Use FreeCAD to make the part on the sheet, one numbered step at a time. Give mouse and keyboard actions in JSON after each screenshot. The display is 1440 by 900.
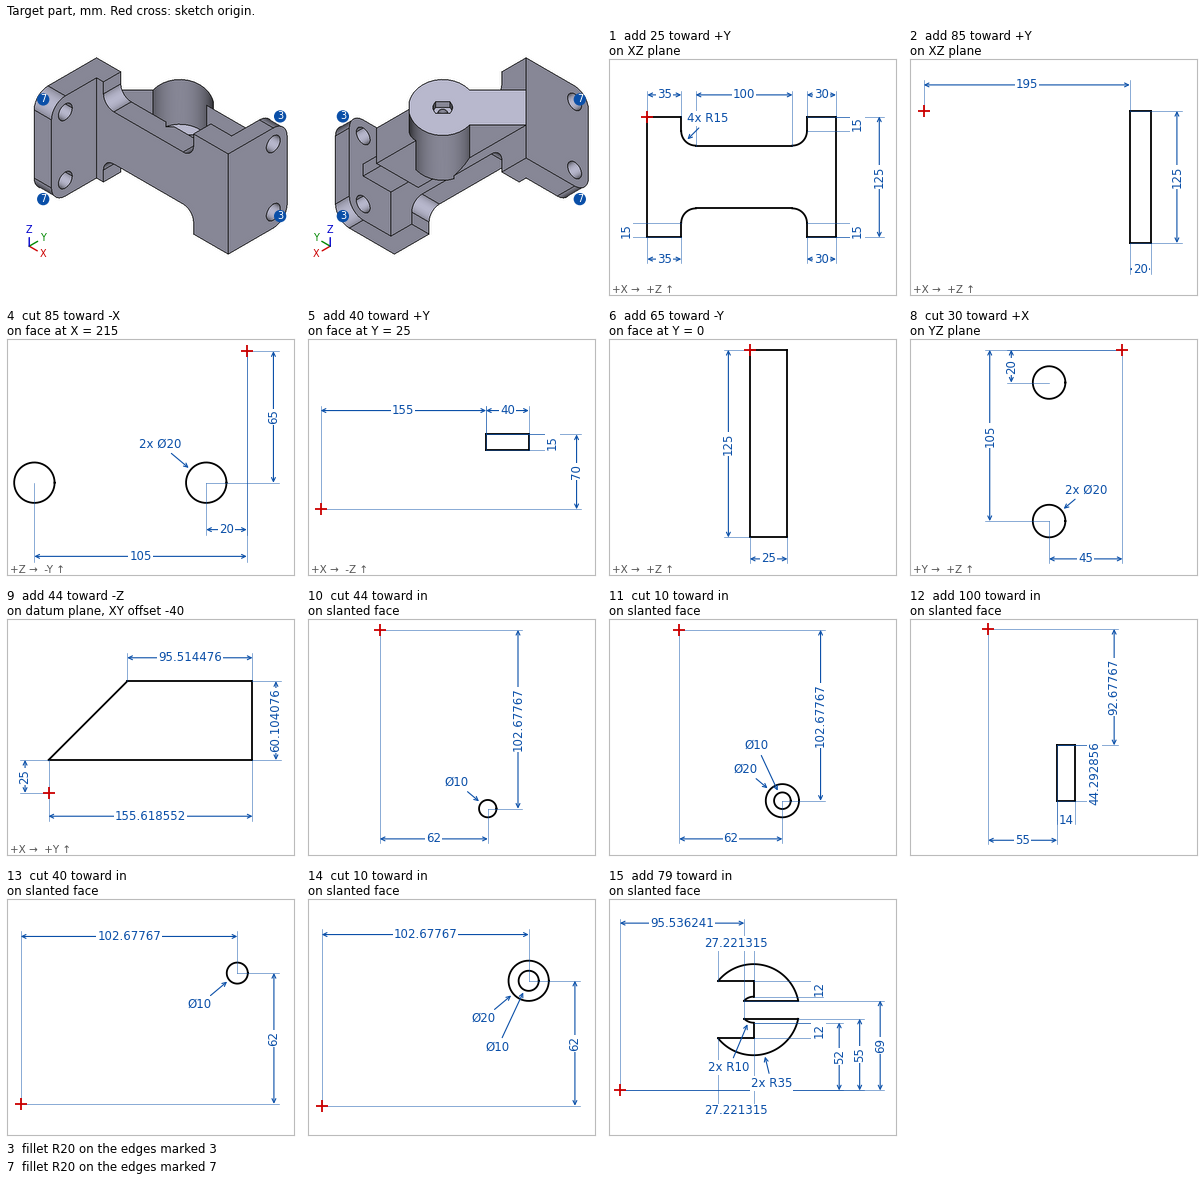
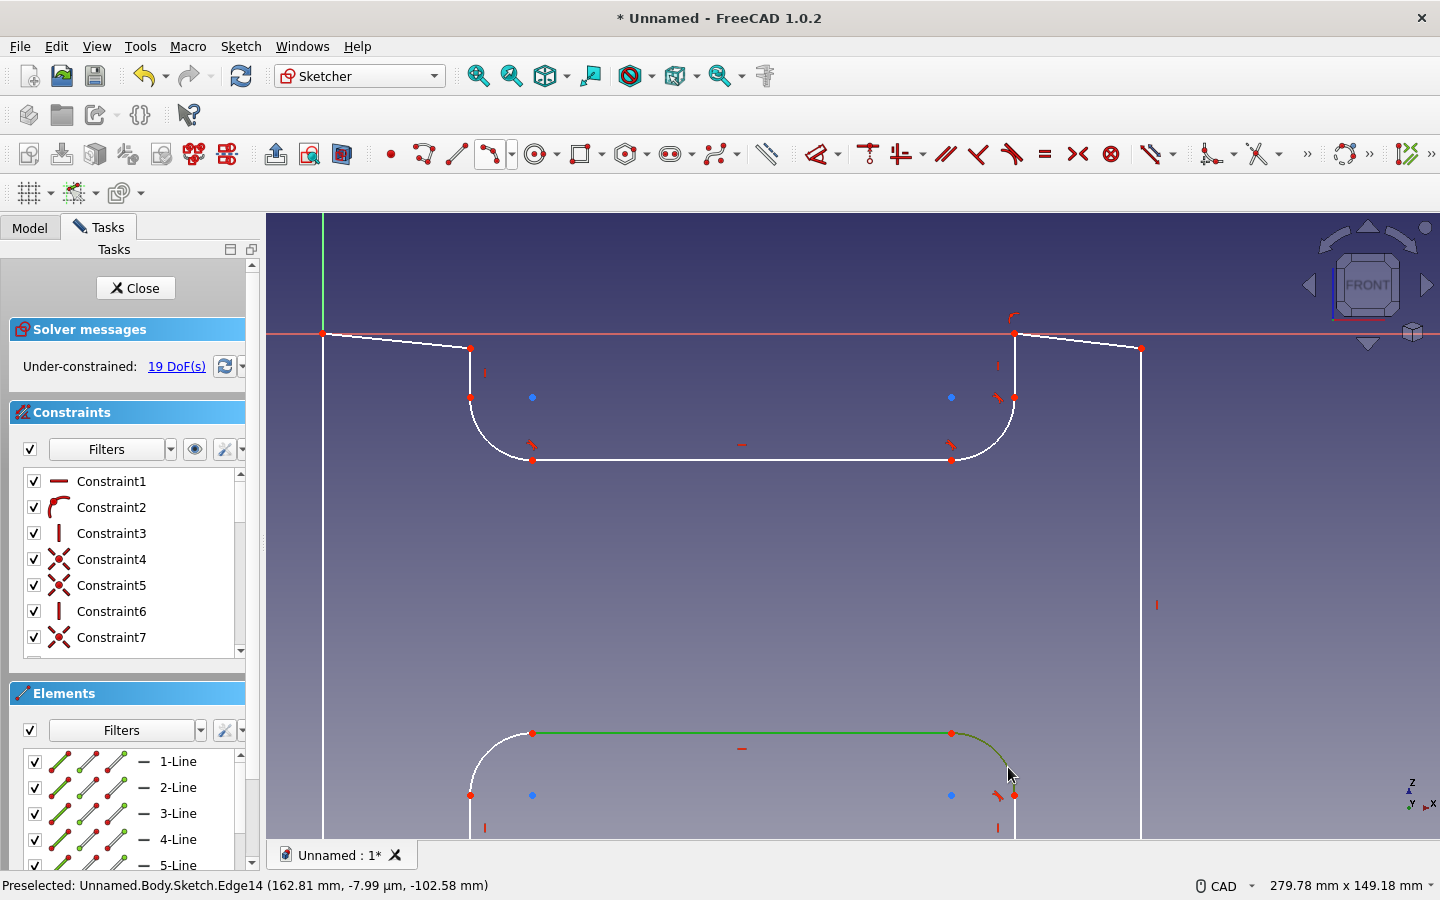
{"action": "left_click", "coordinate": [1012, 154]}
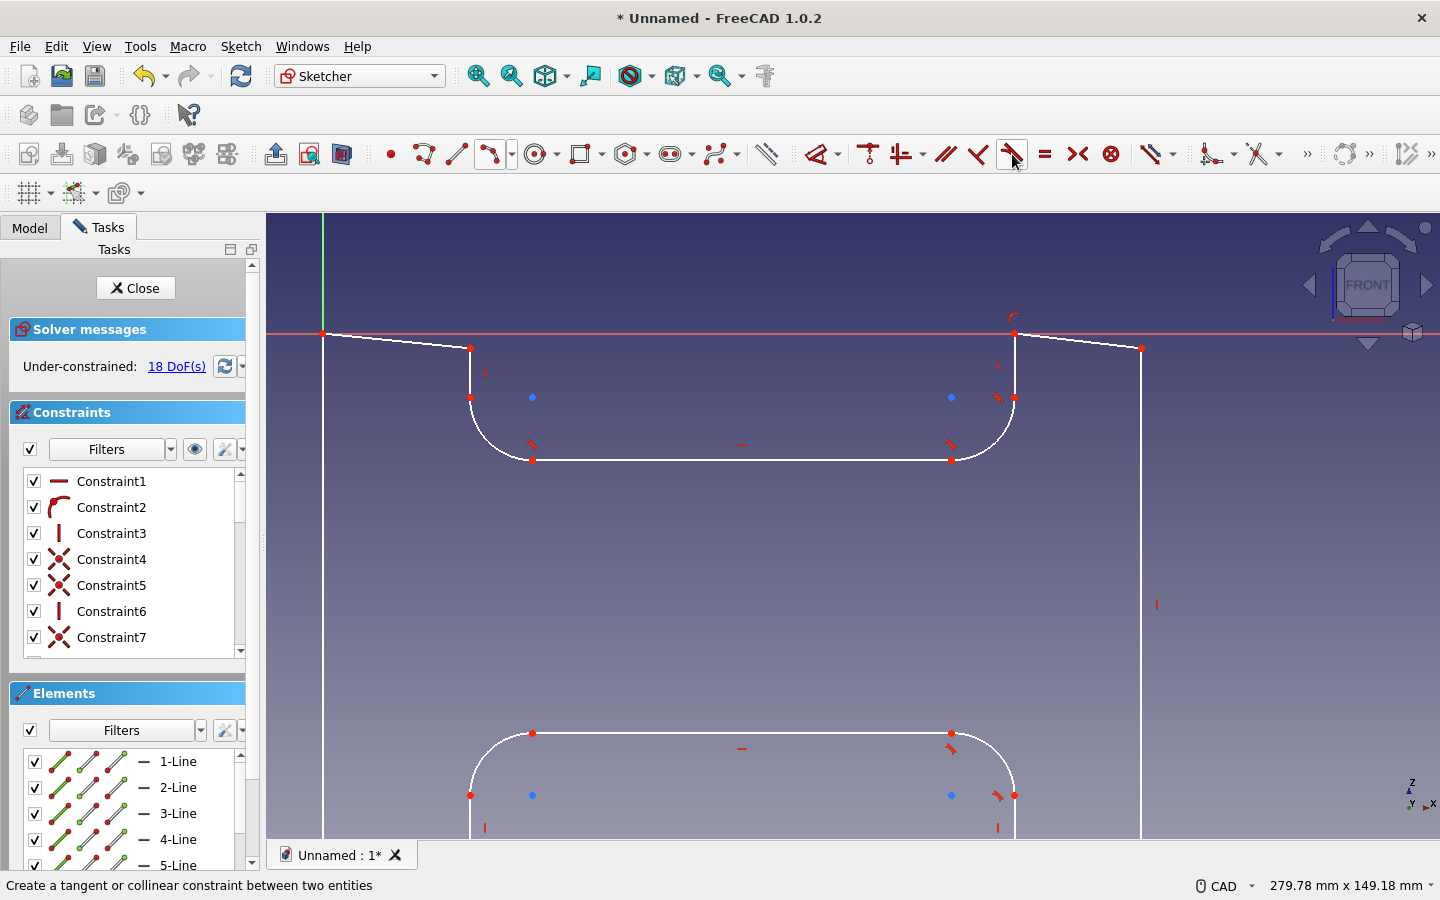
{"action": "left_click", "coordinate": [826, 733]}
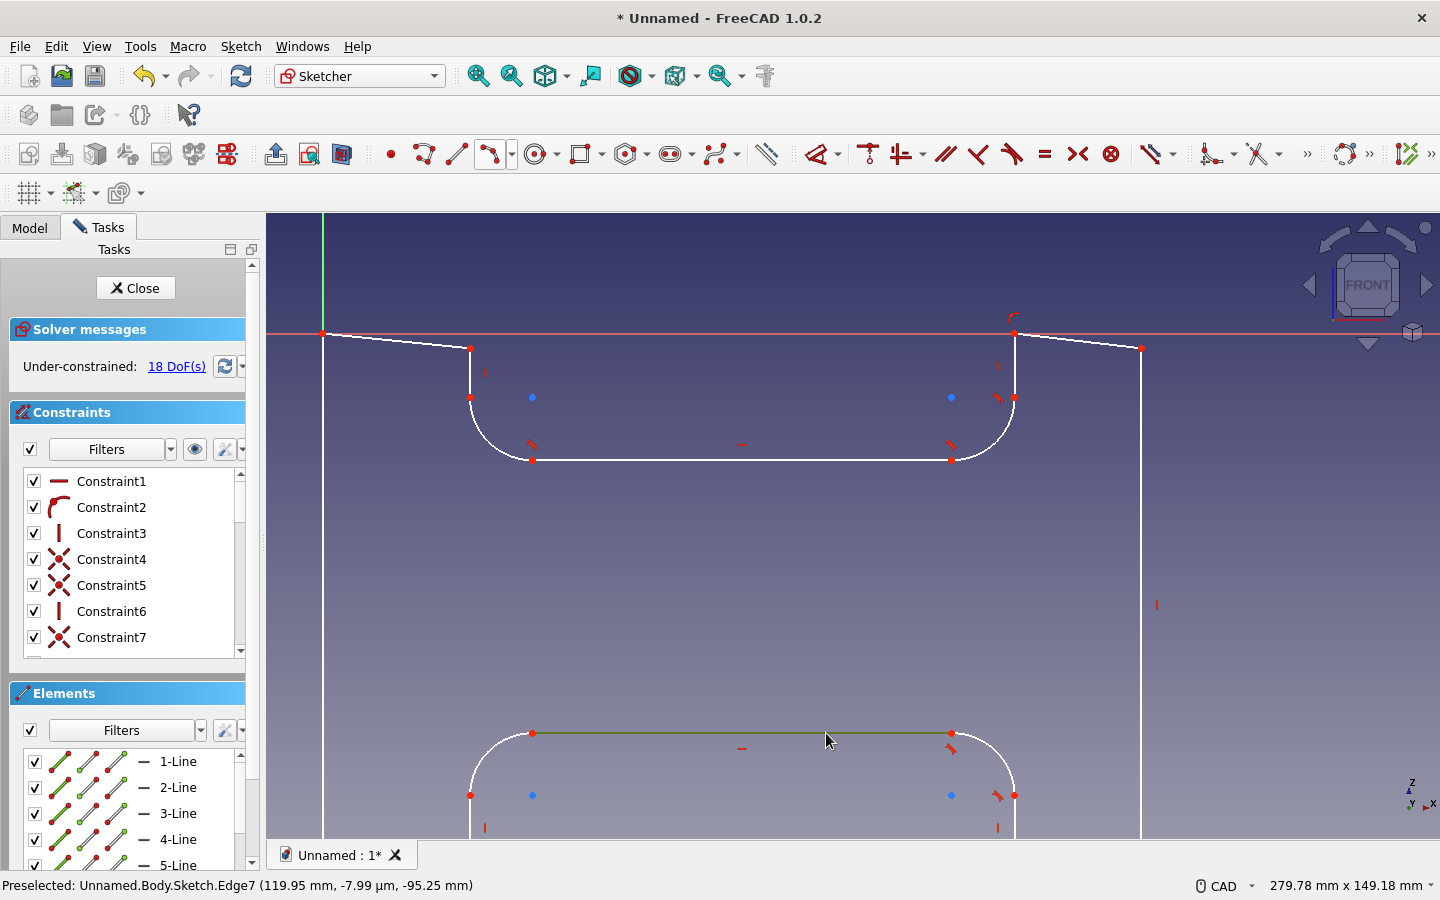
{"action": "left_click", "coordinate": [504, 740]}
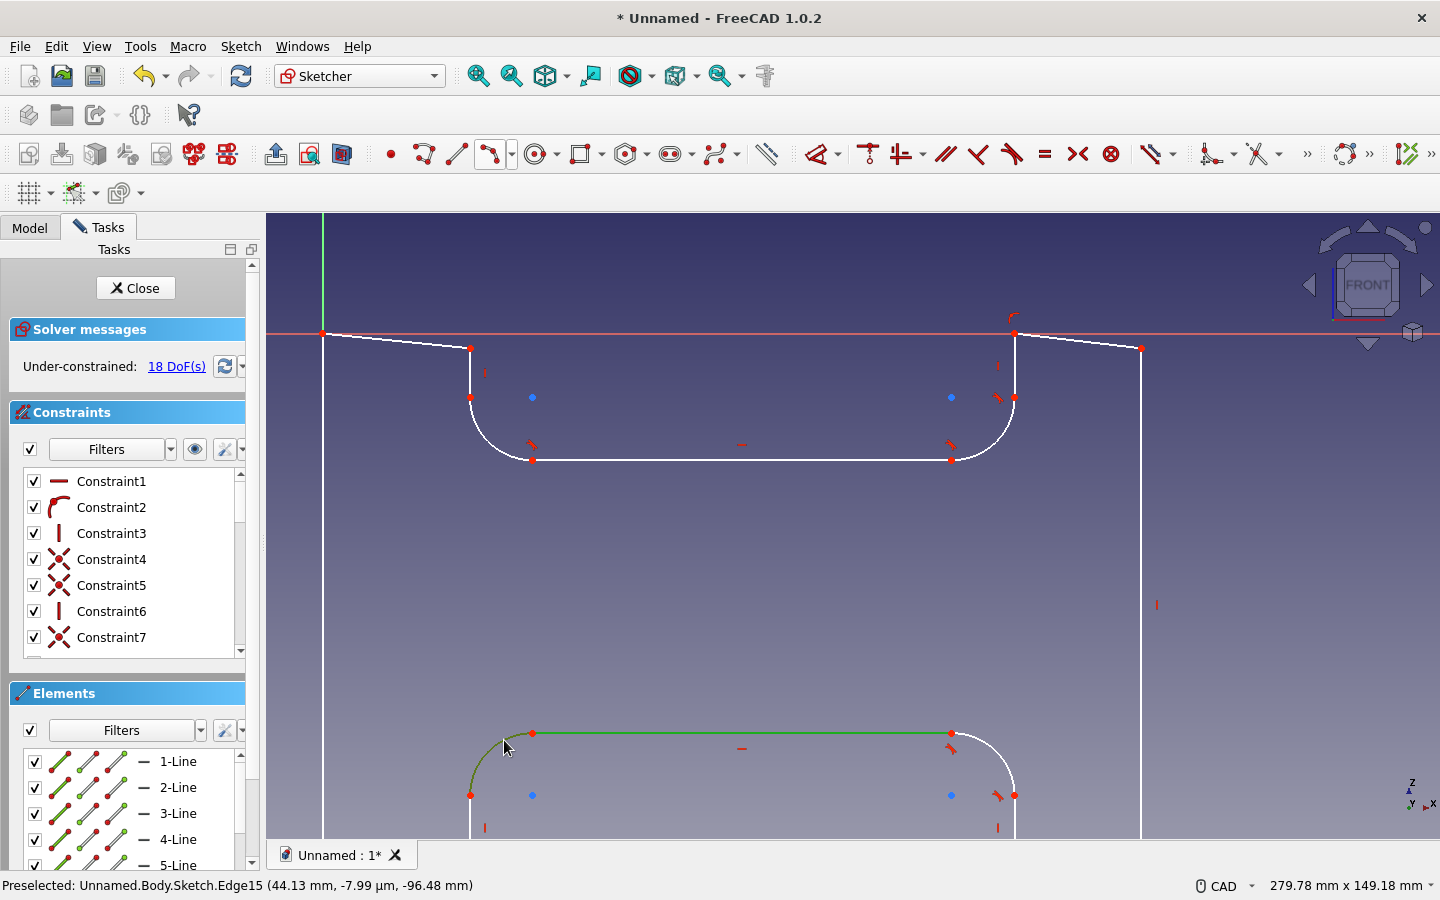
{"action": "left_click", "coordinate": [1012, 154]}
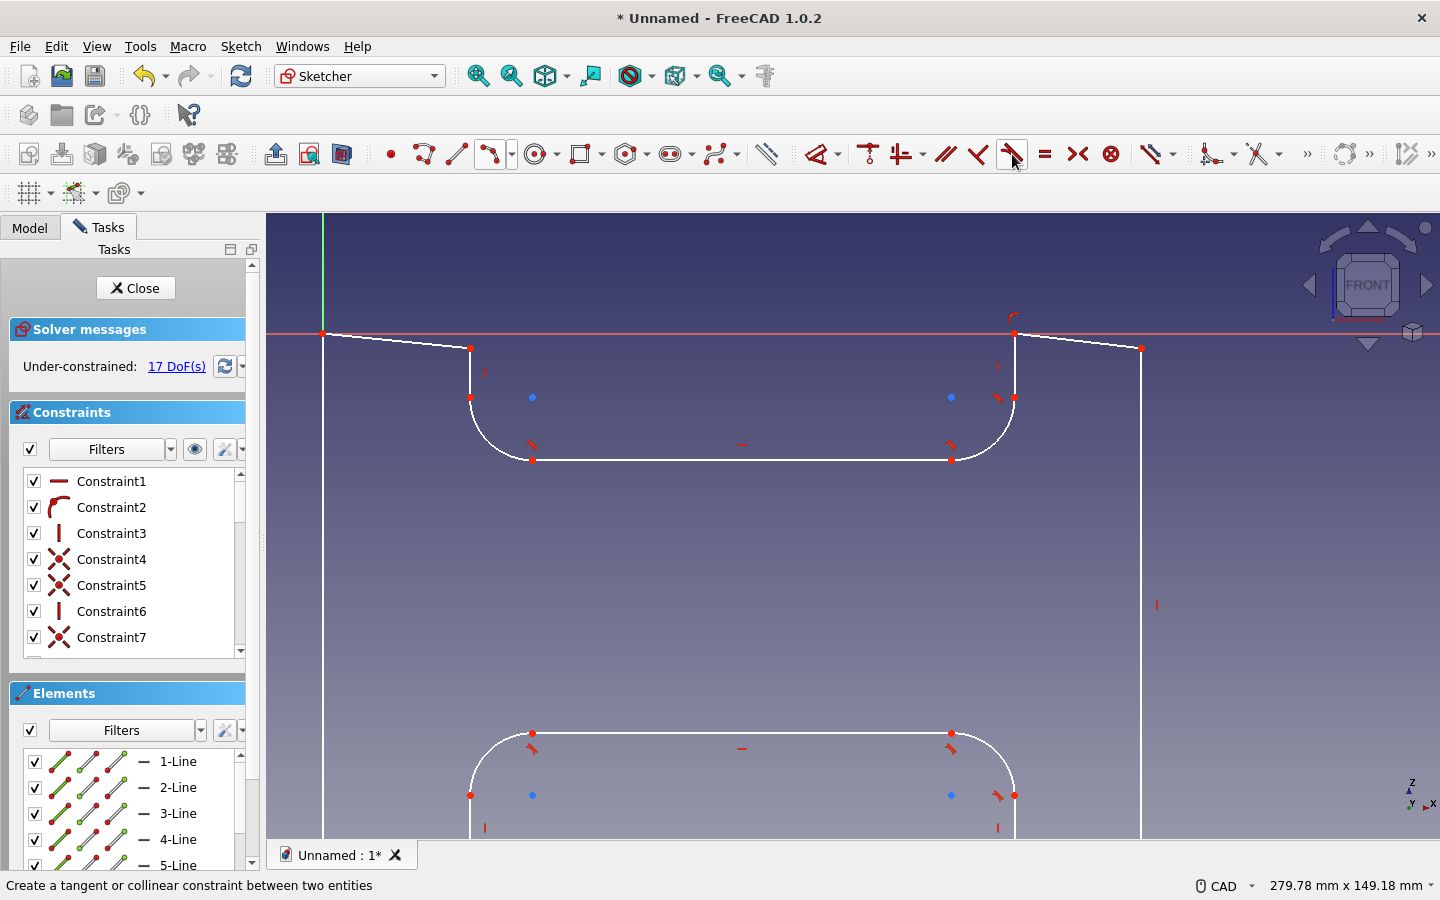
{"action": "left_click", "coordinate": [470, 809]}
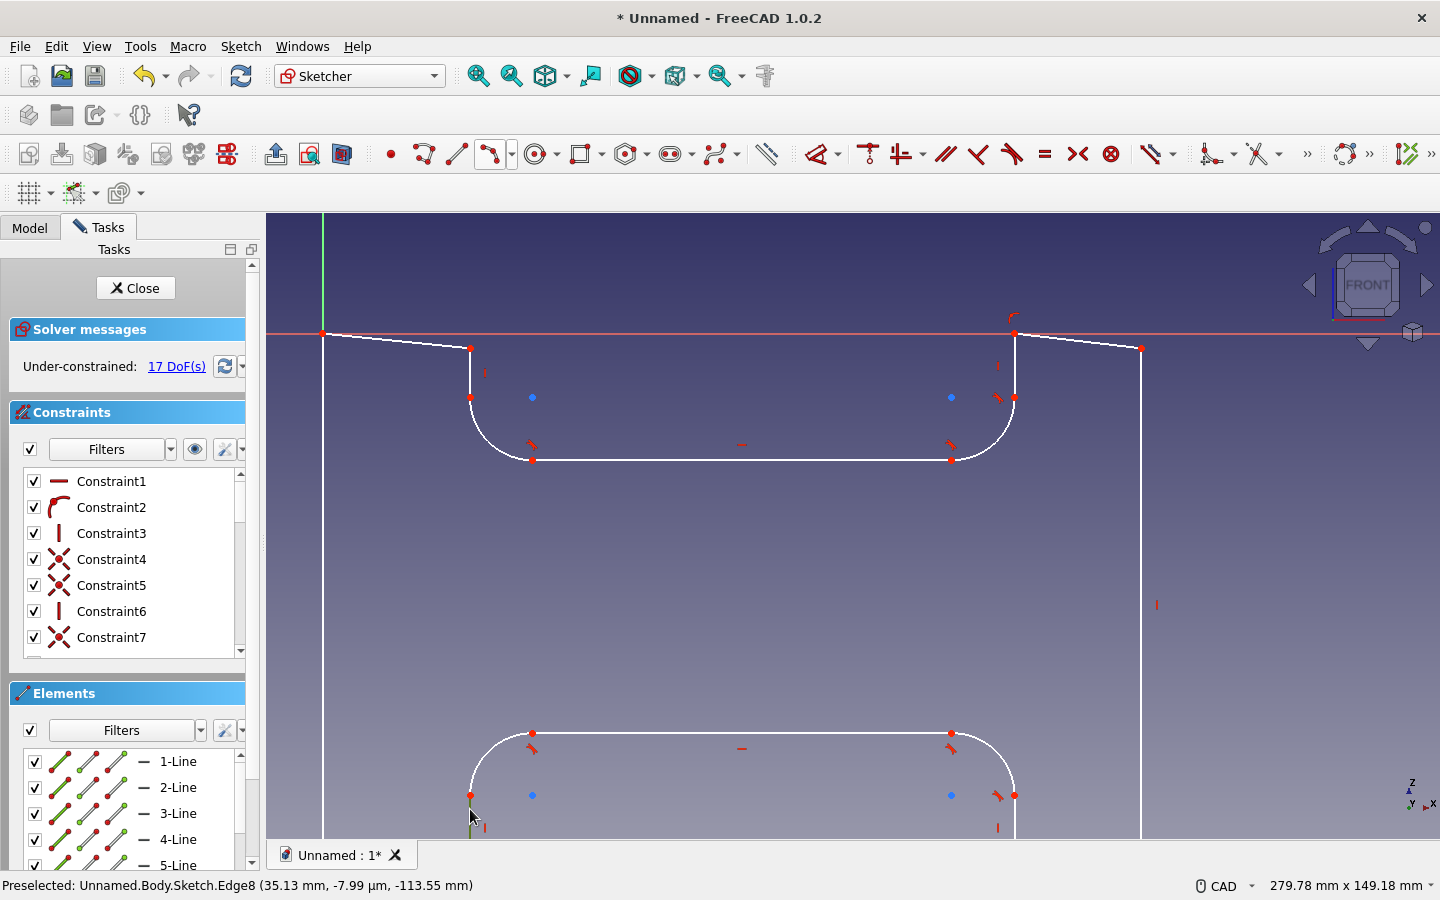
{"action": "left_click", "coordinate": [504, 740]}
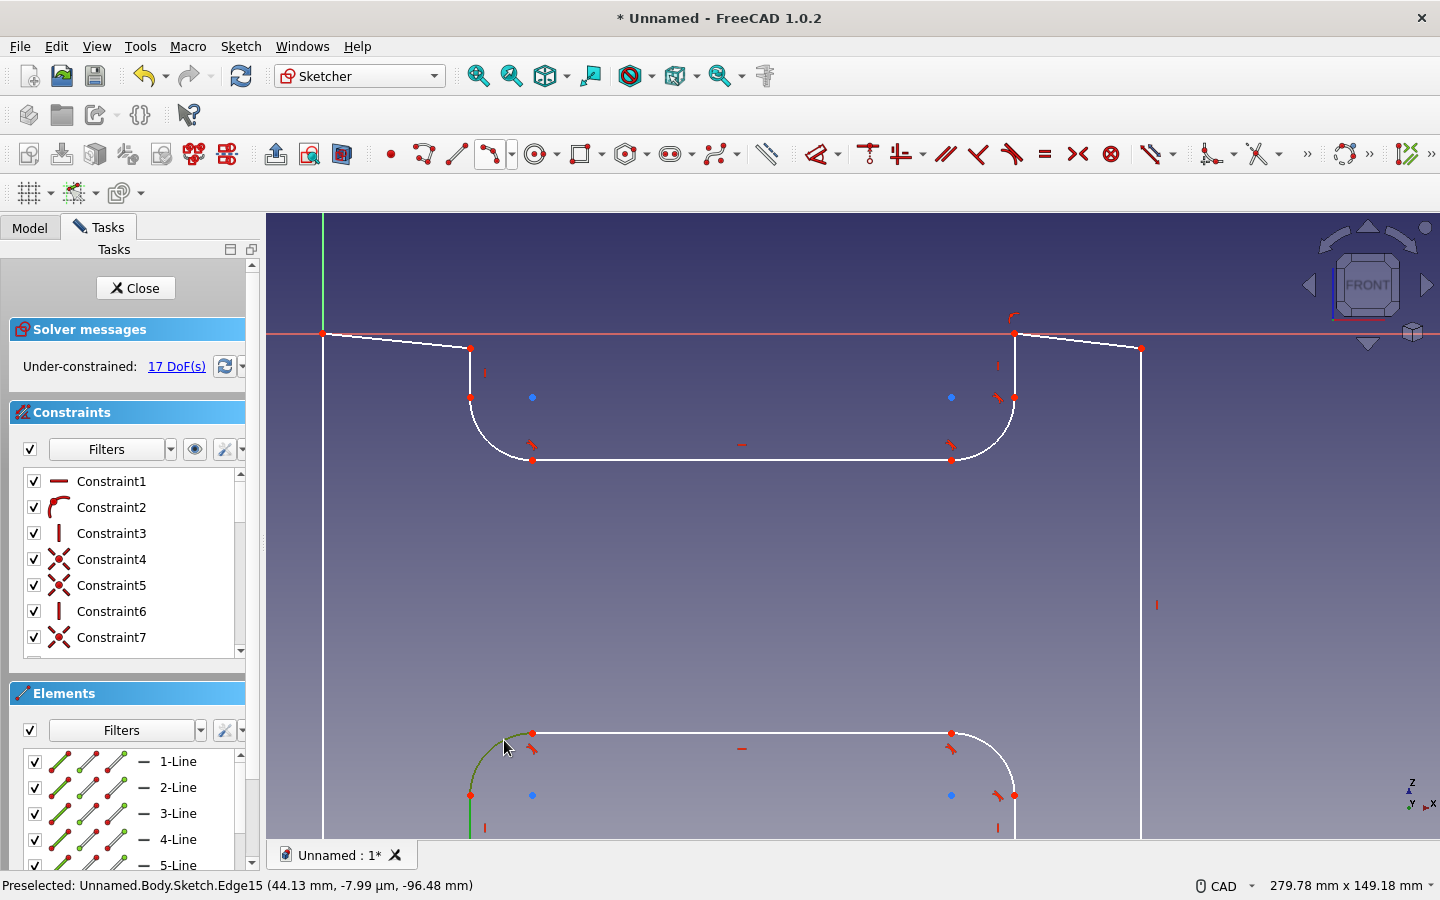
{"action": "key", "text": "t"}